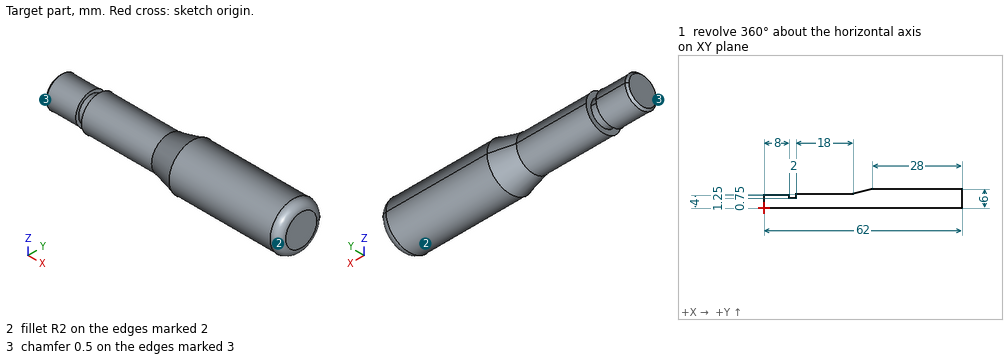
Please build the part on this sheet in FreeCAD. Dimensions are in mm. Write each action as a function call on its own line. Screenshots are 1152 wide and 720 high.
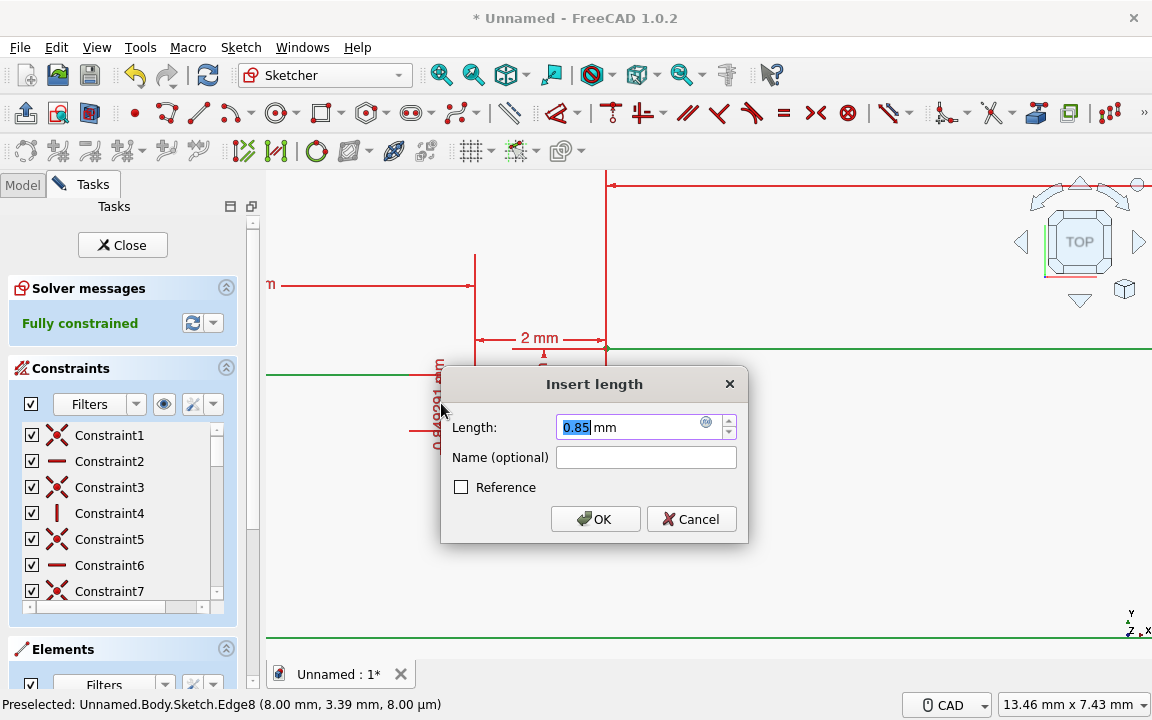
text(0.75)
key(Return)
key(Escape)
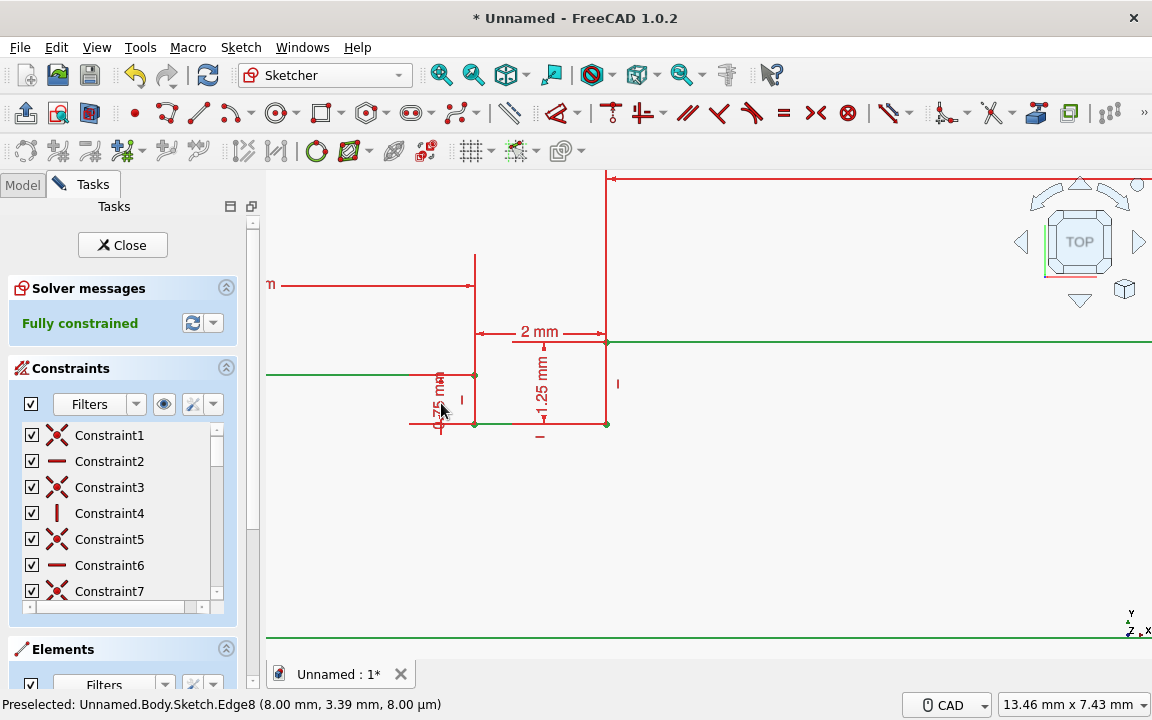
click(123, 245)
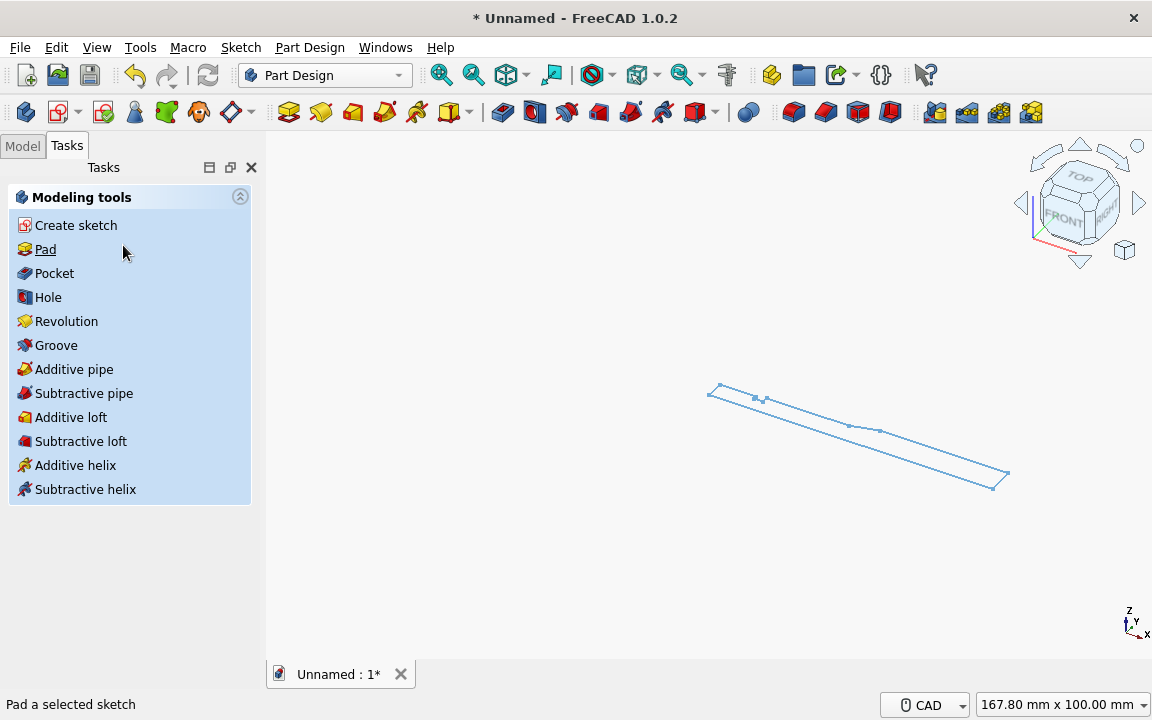
click(322, 112)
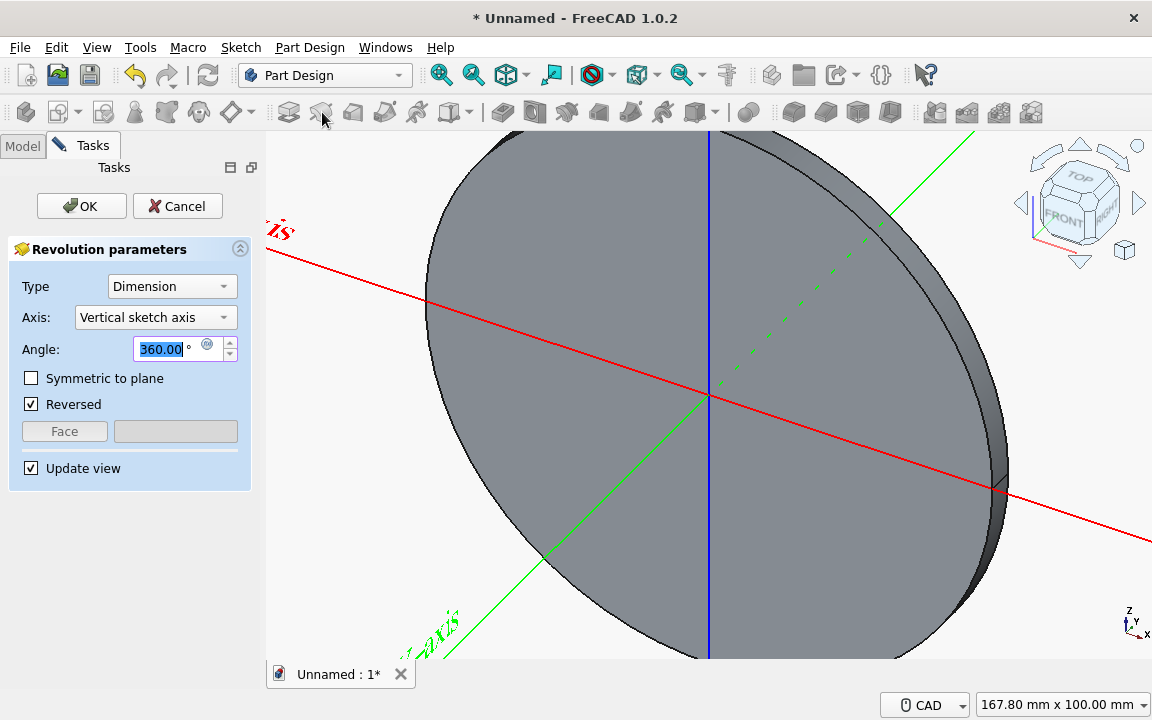
click(156, 318)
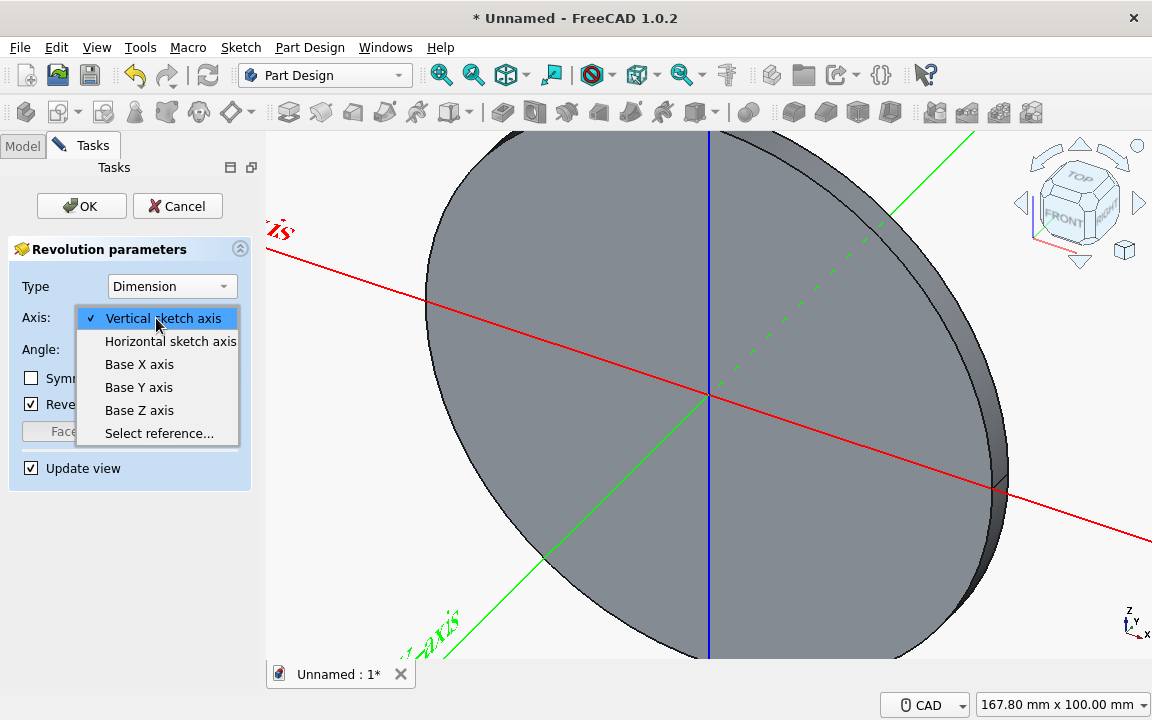
click(156, 342)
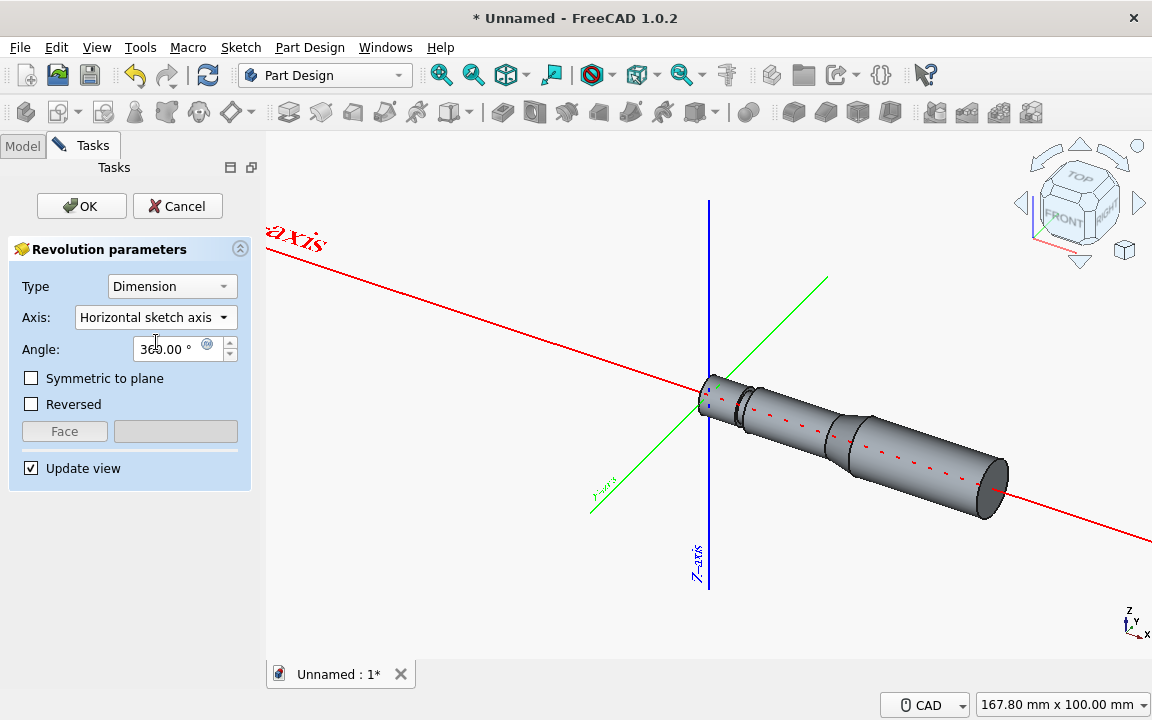
click(82, 206)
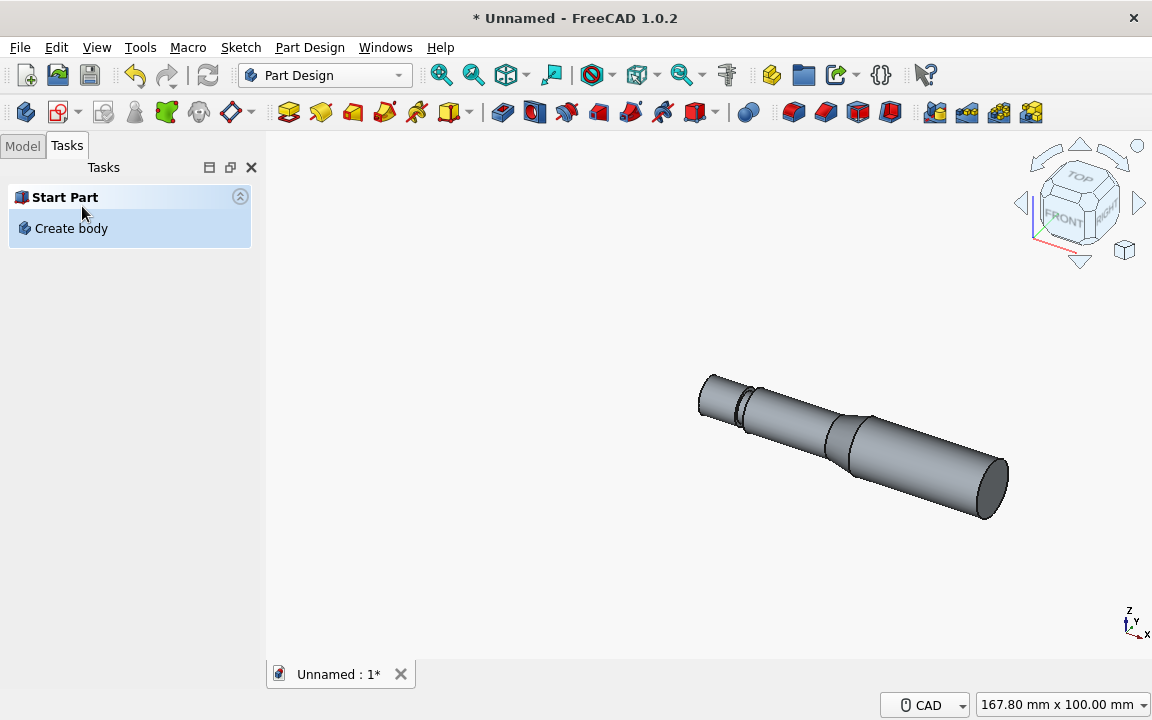
click(442, 76)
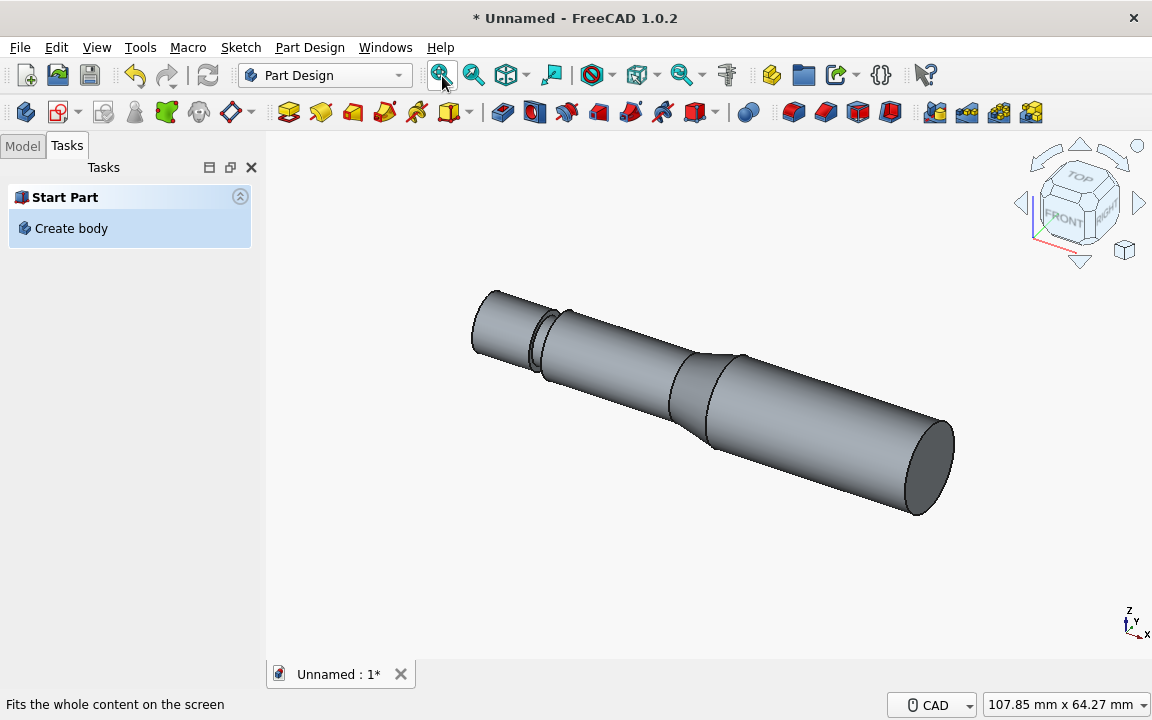
click(905, 492)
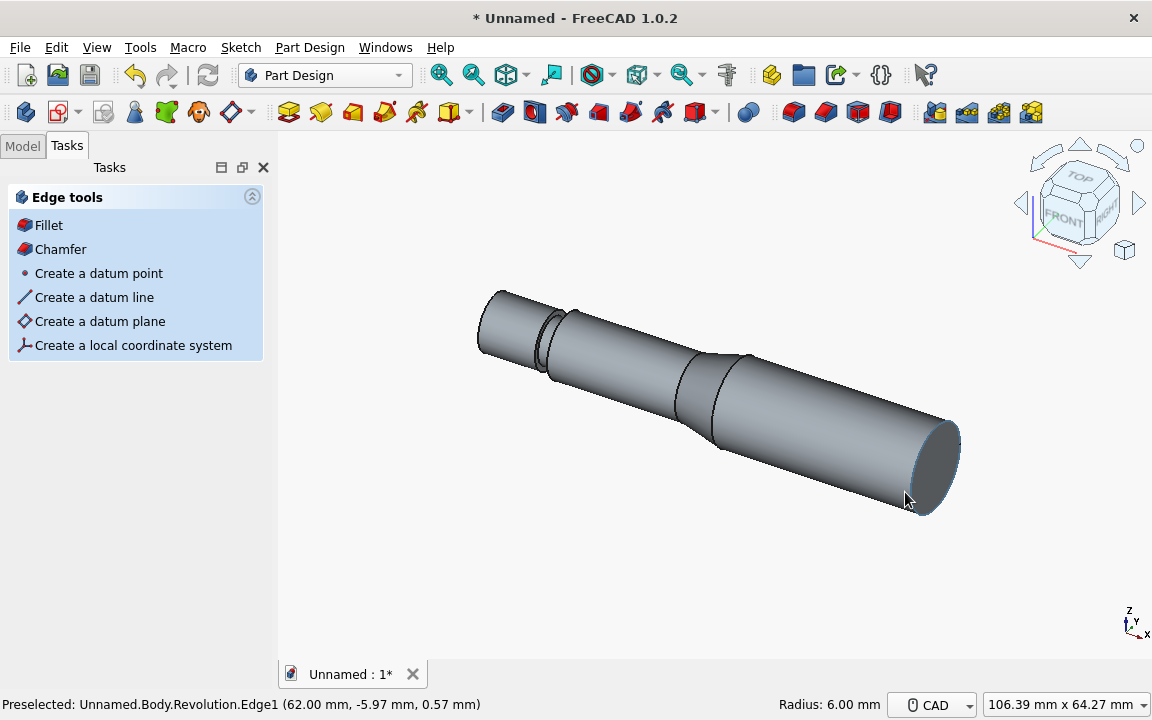
click(794, 112)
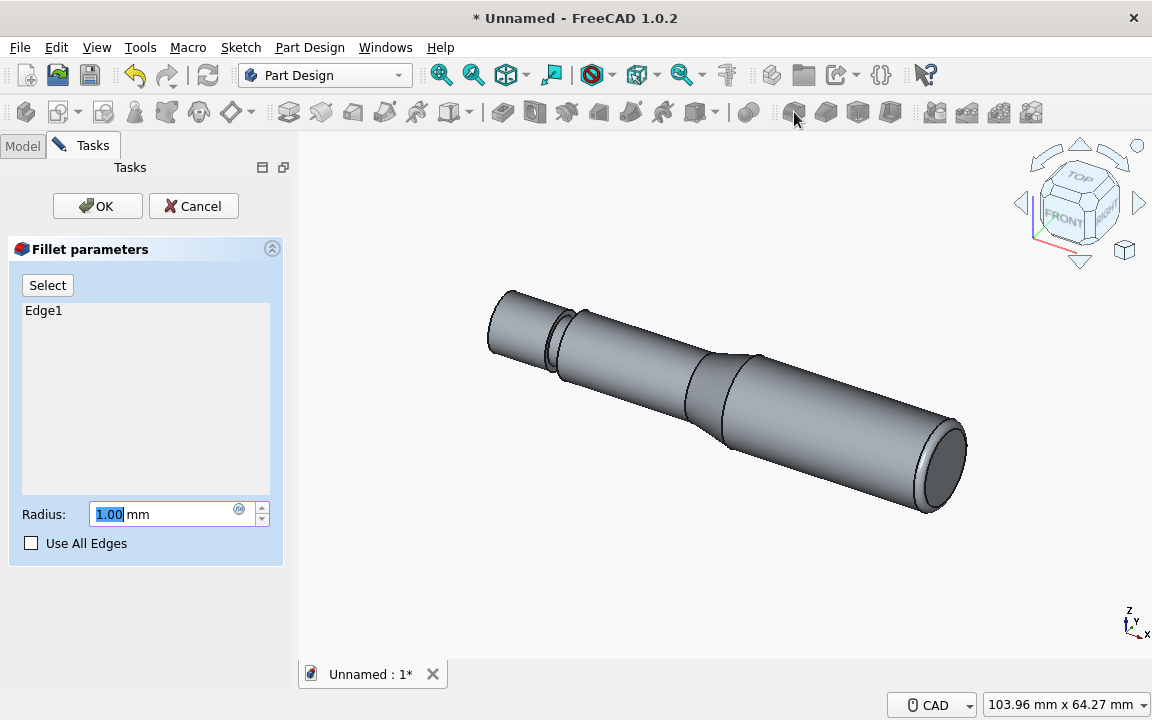
text(2)
key(Tab)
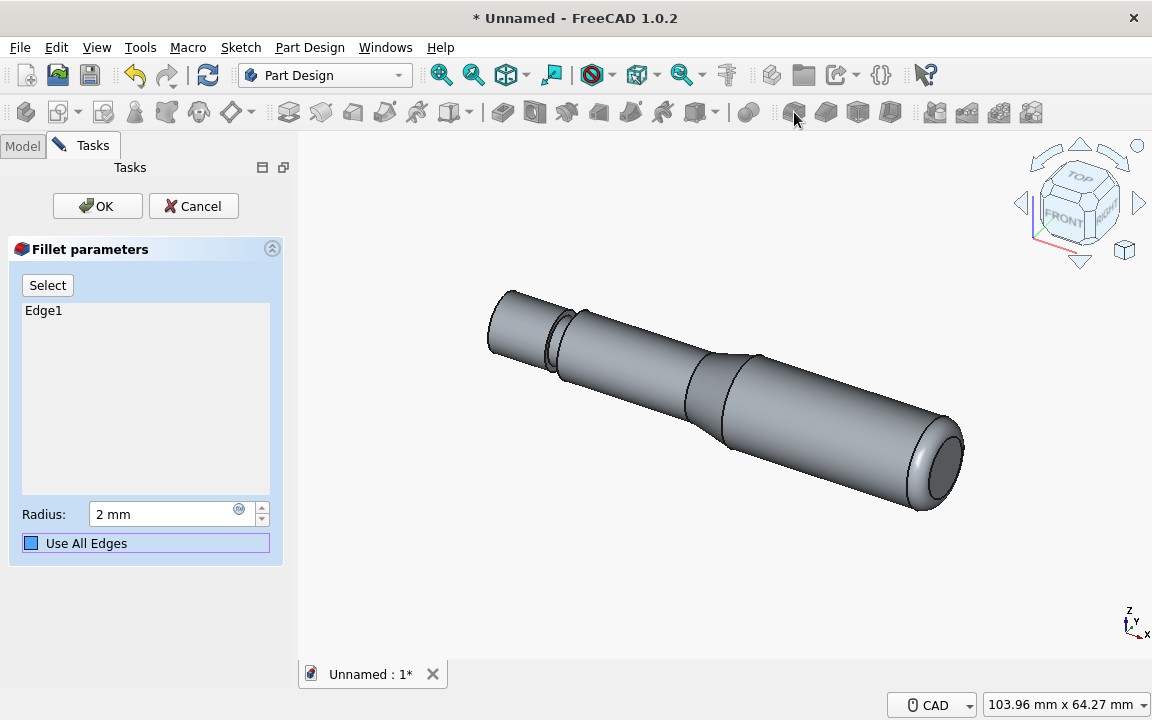
click(98, 206)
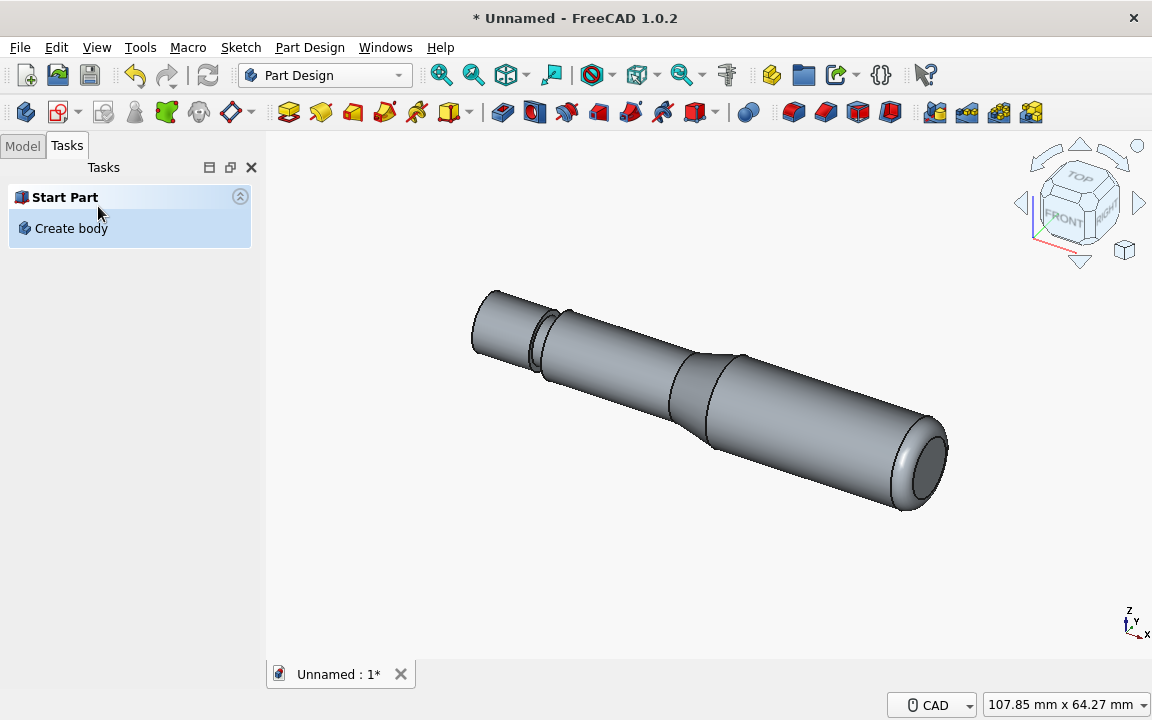
click(472, 337)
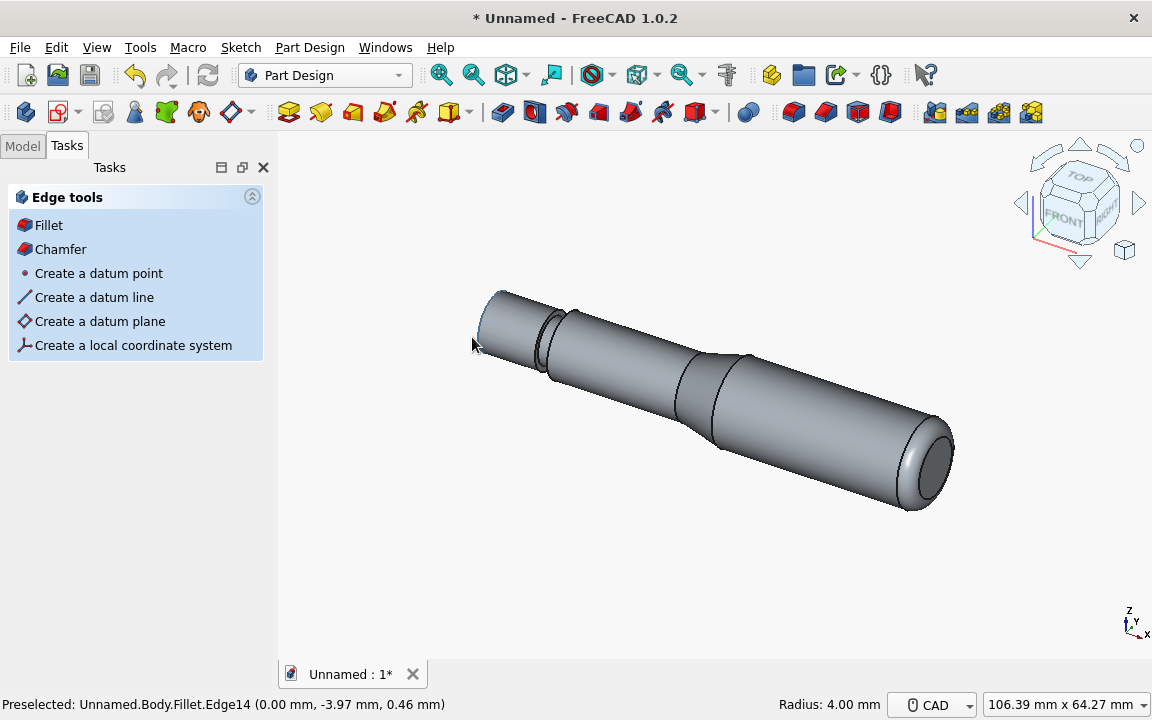
click(826, 112)